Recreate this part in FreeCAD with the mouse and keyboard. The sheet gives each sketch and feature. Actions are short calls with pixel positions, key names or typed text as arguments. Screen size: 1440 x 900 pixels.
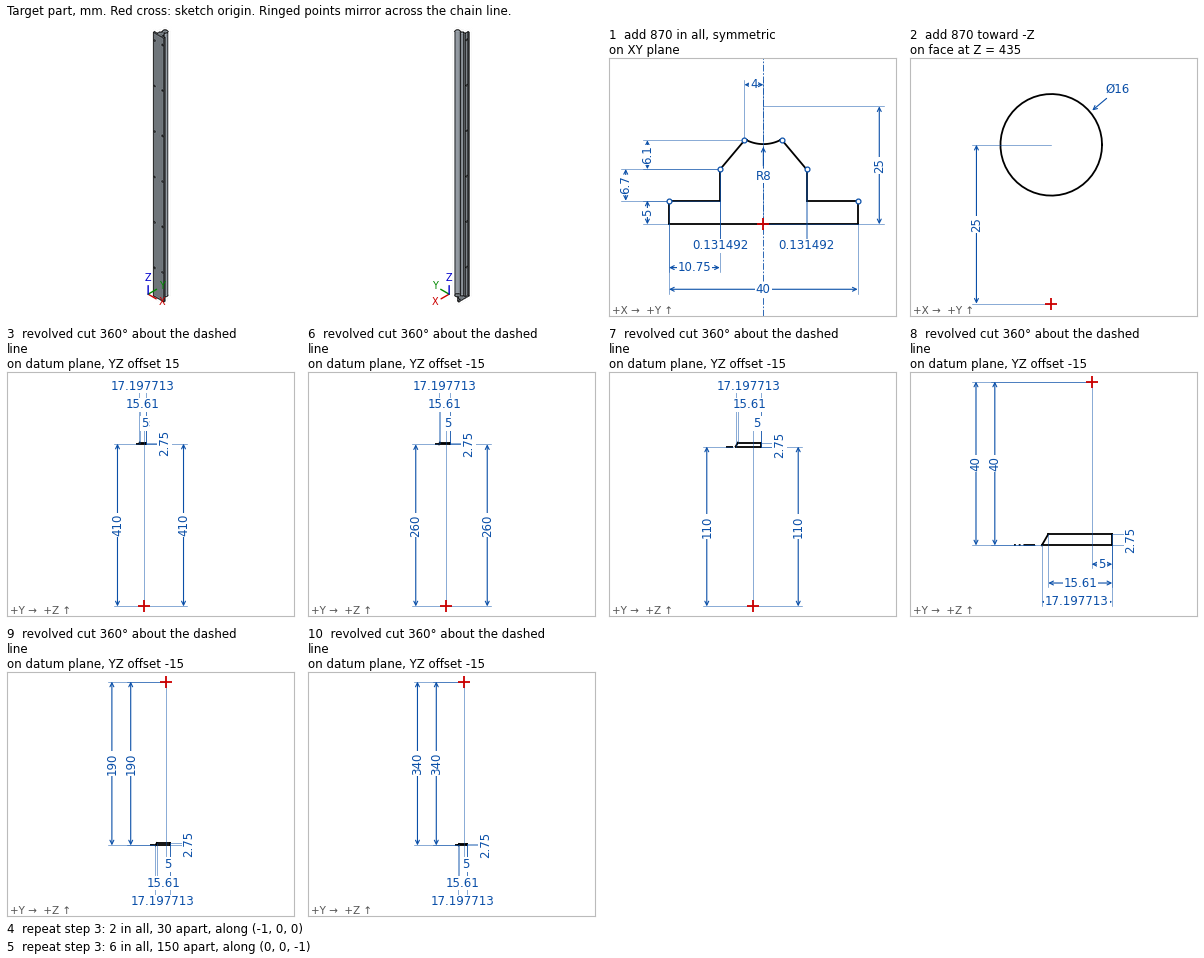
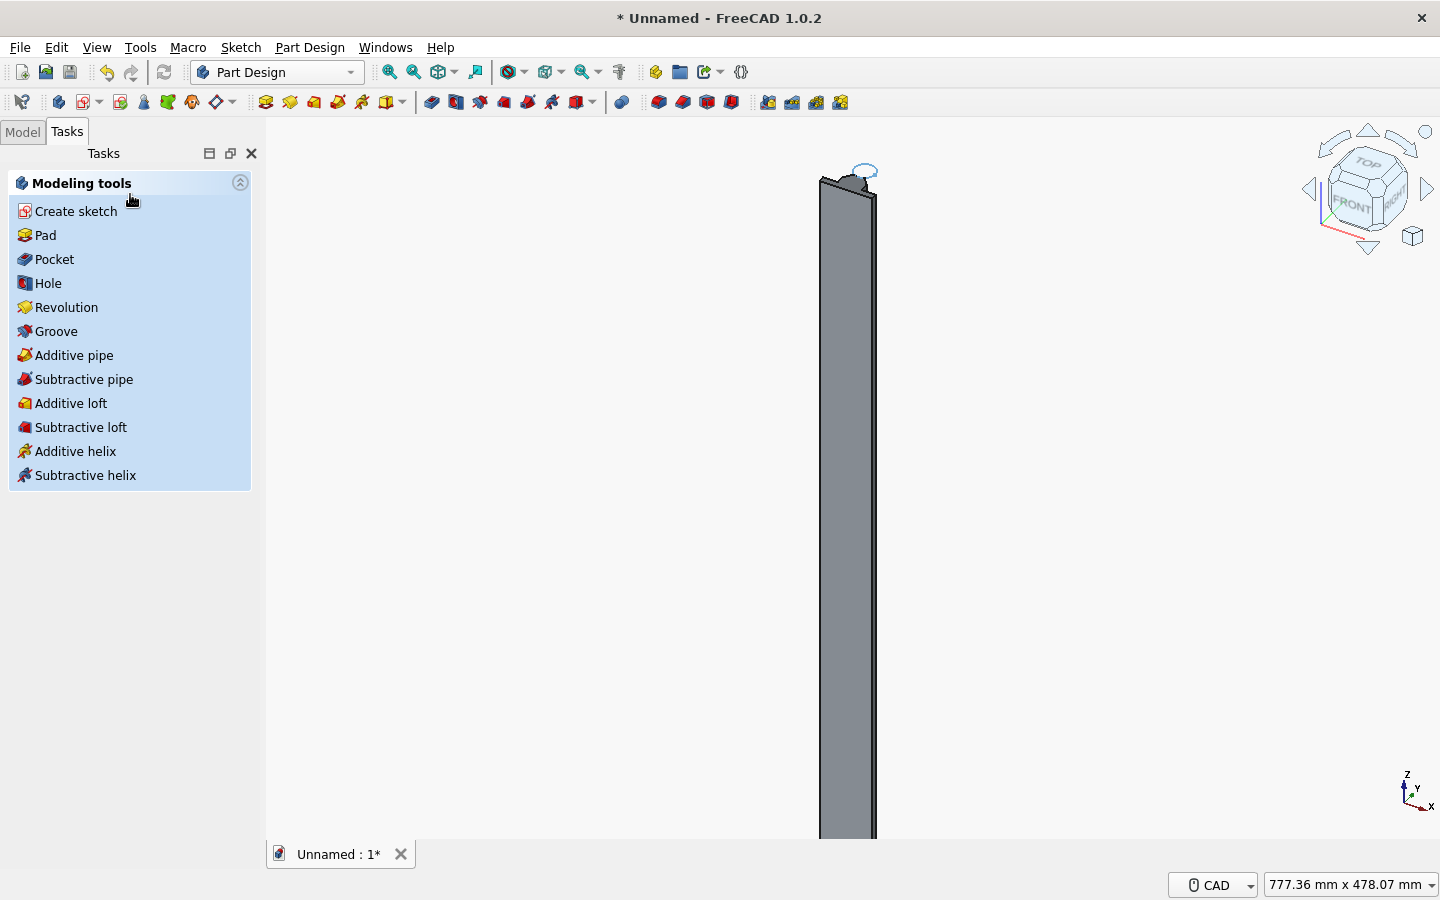
click(266, 102)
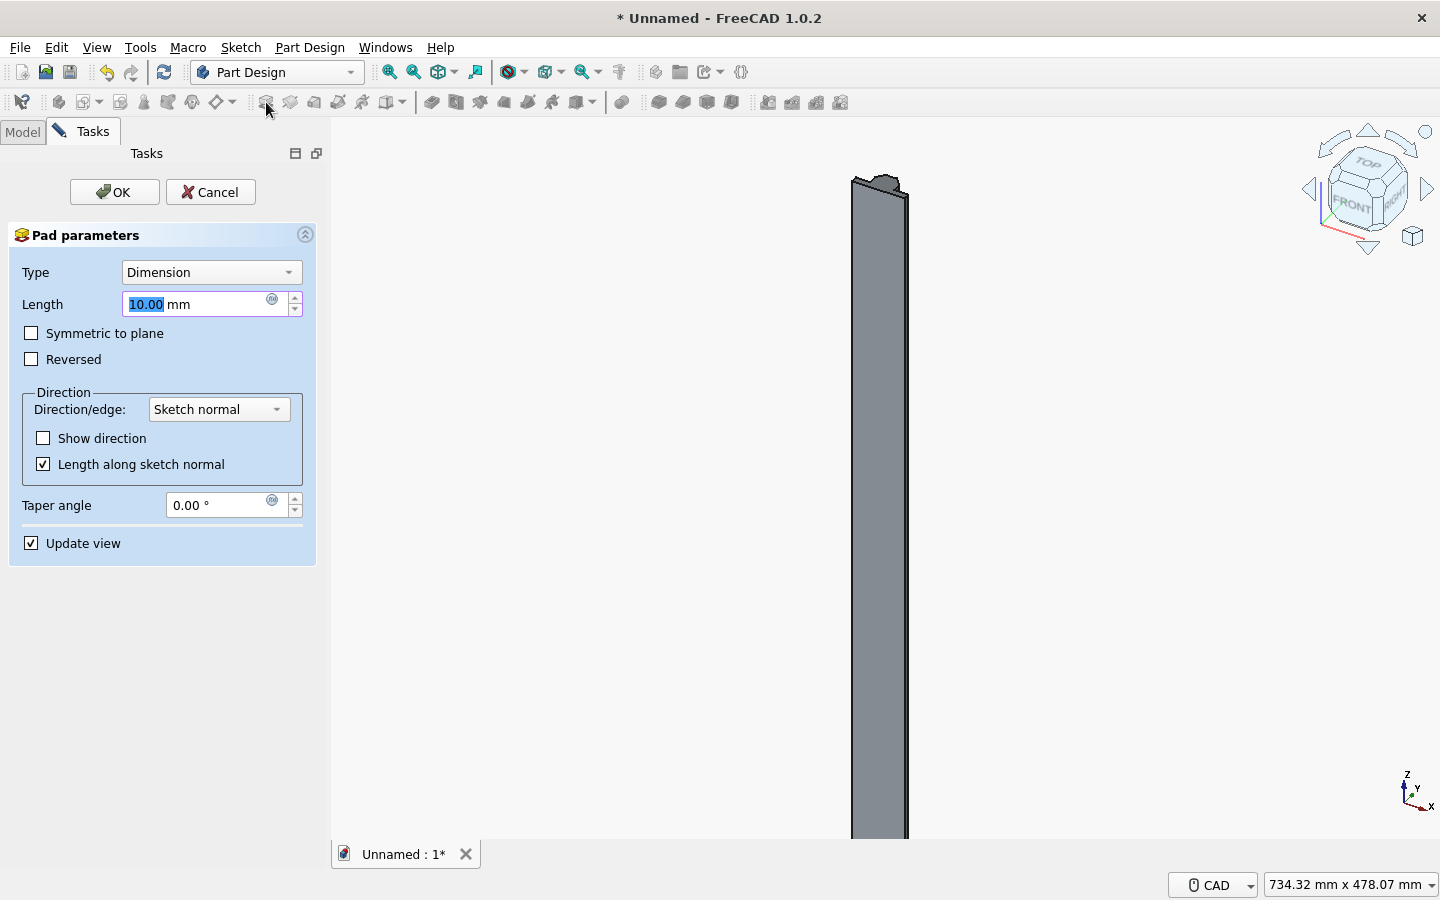
text(870)
key(Tab)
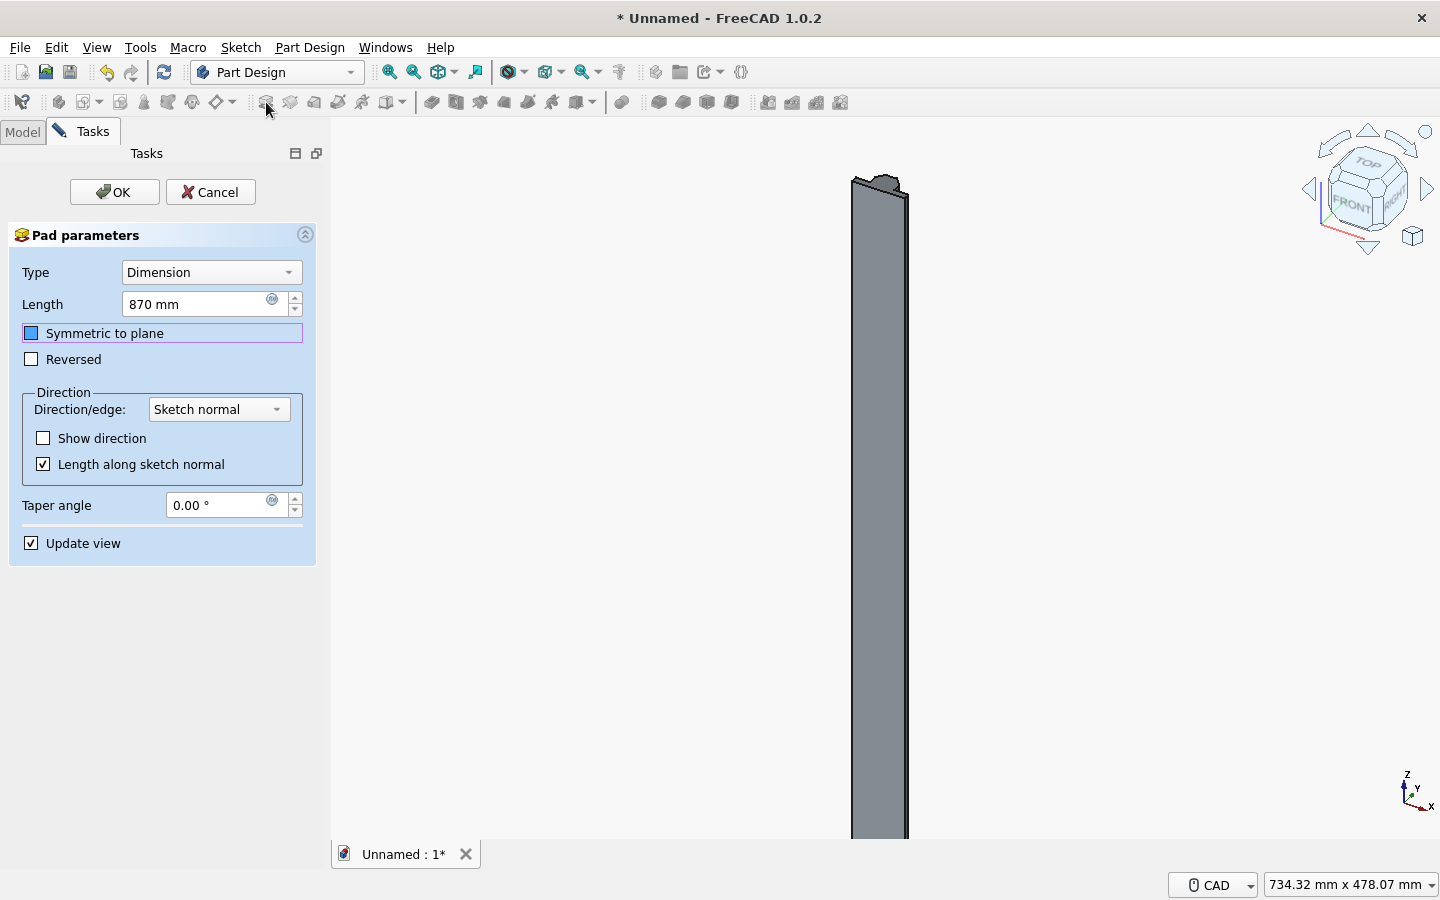
click(30, 359)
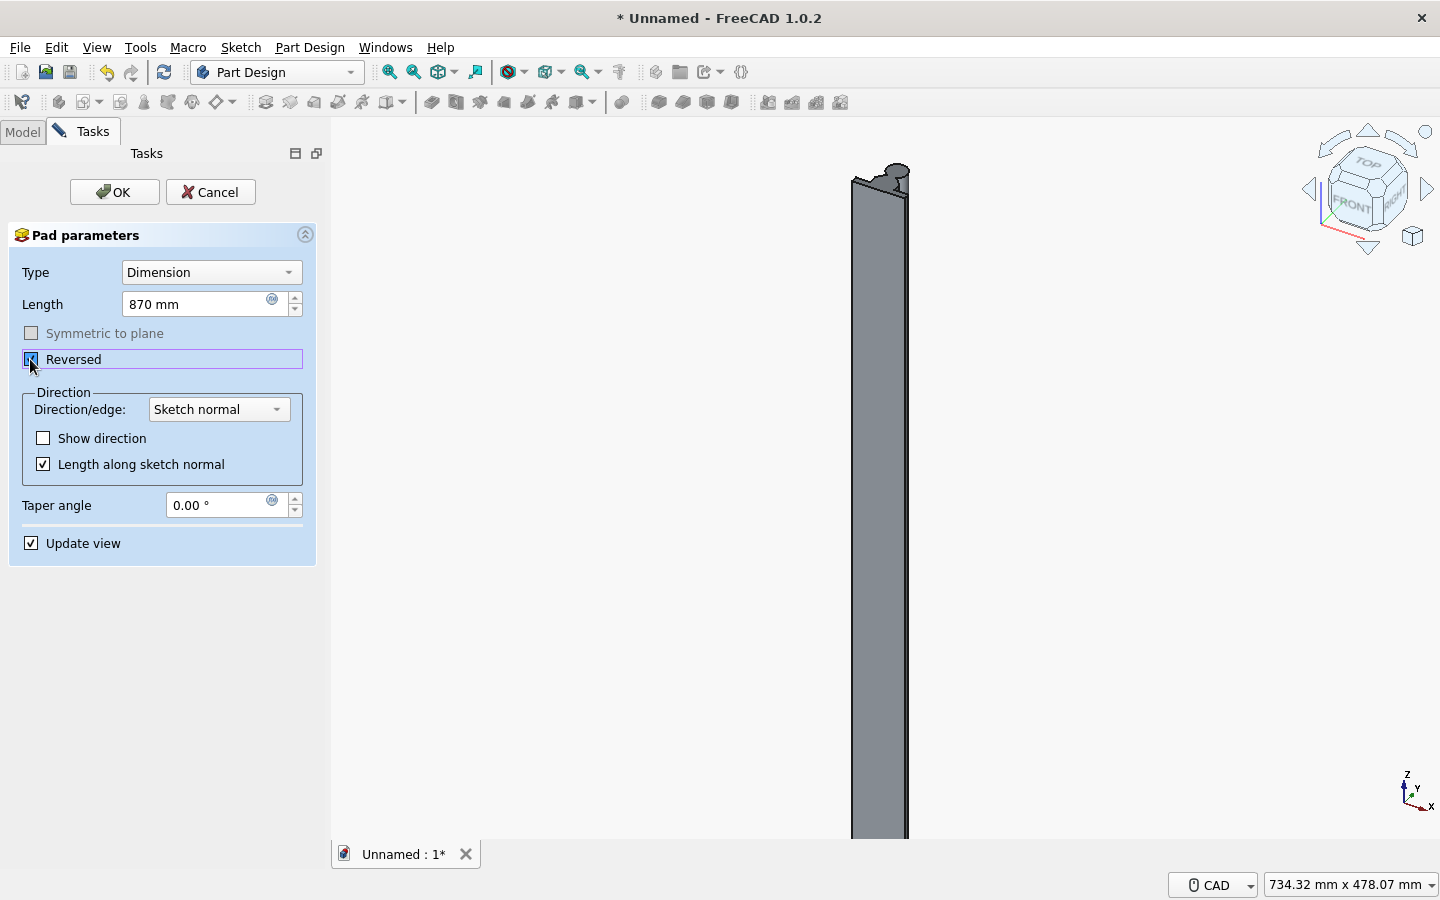
click(115, 192)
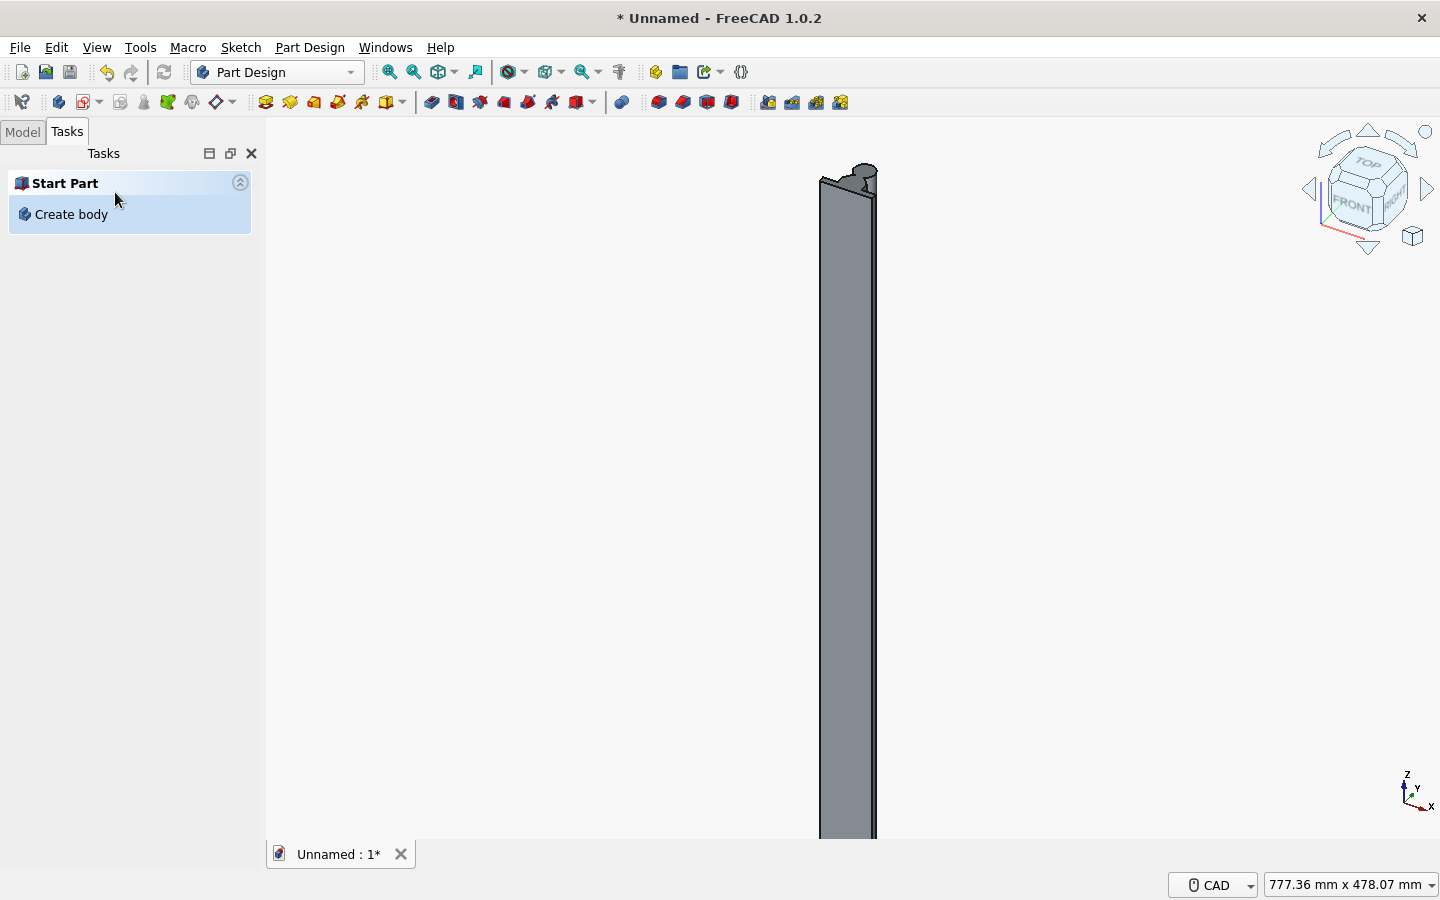
key(v)
key(f)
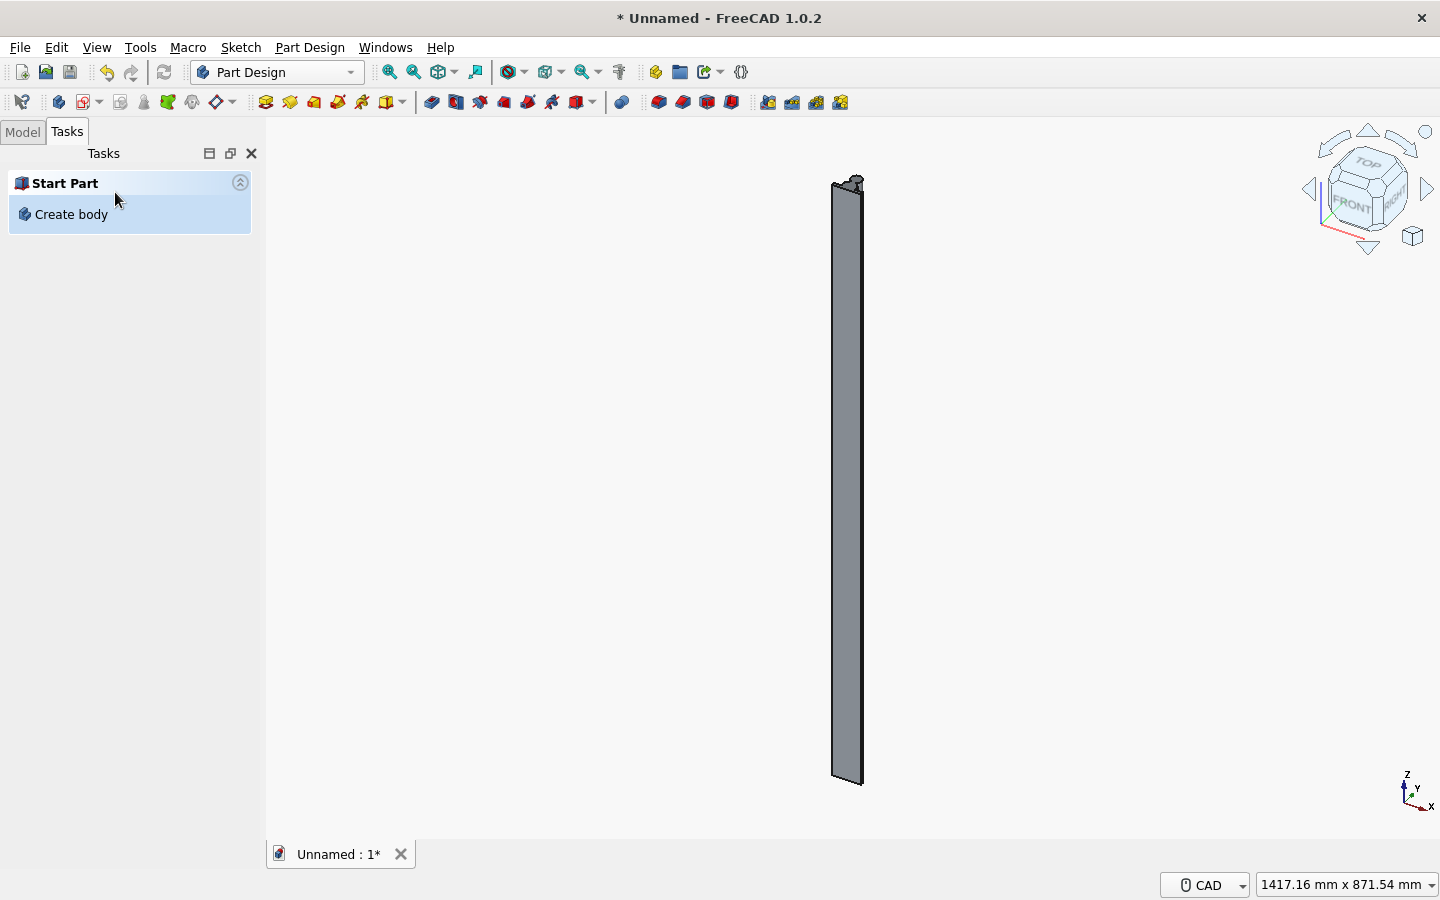
click(23, 131)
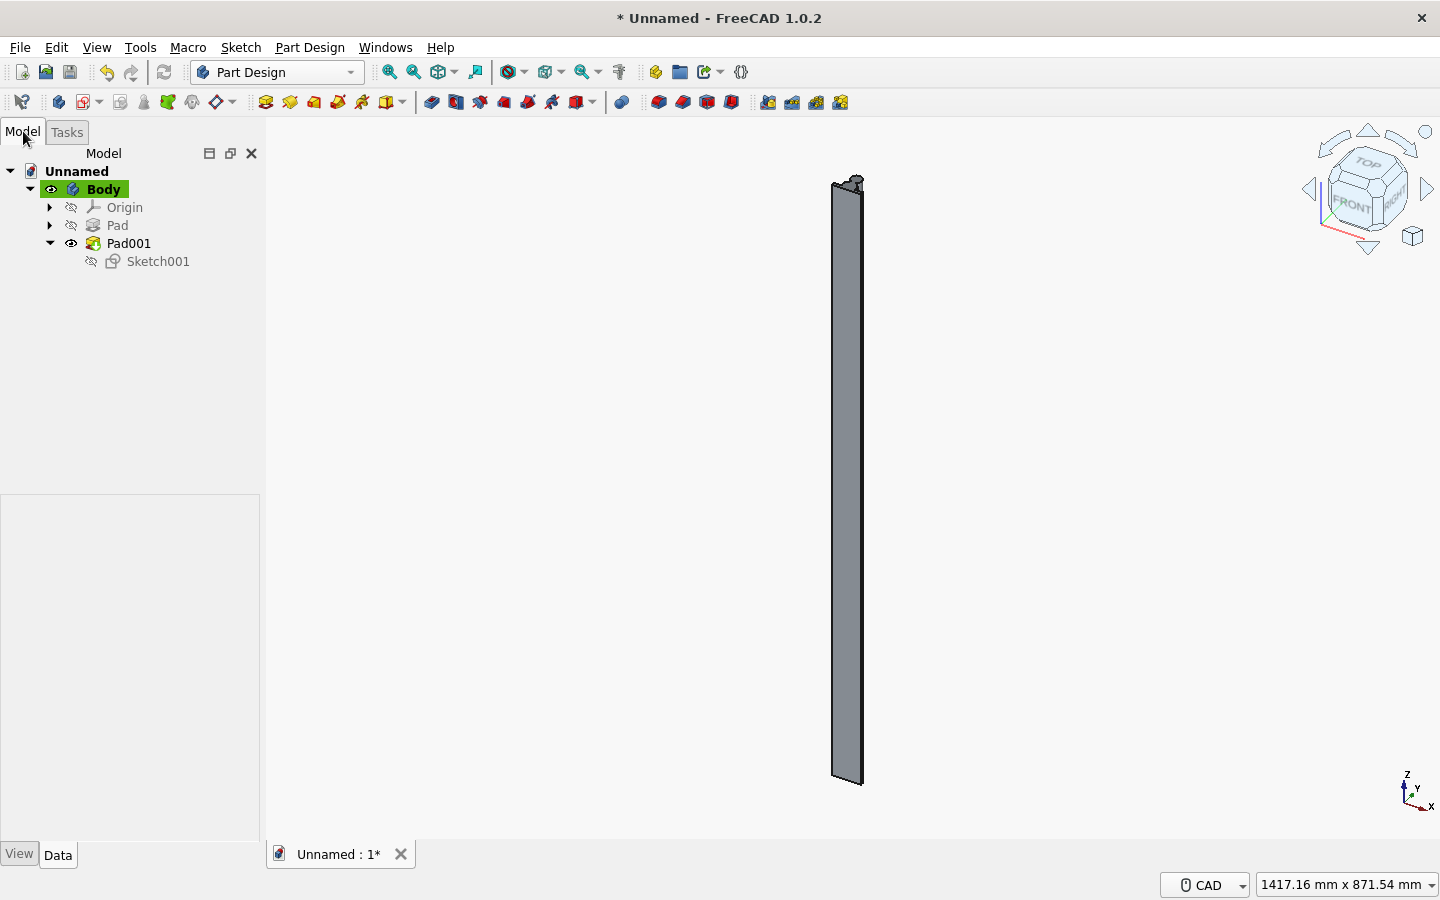
click(50, 207)